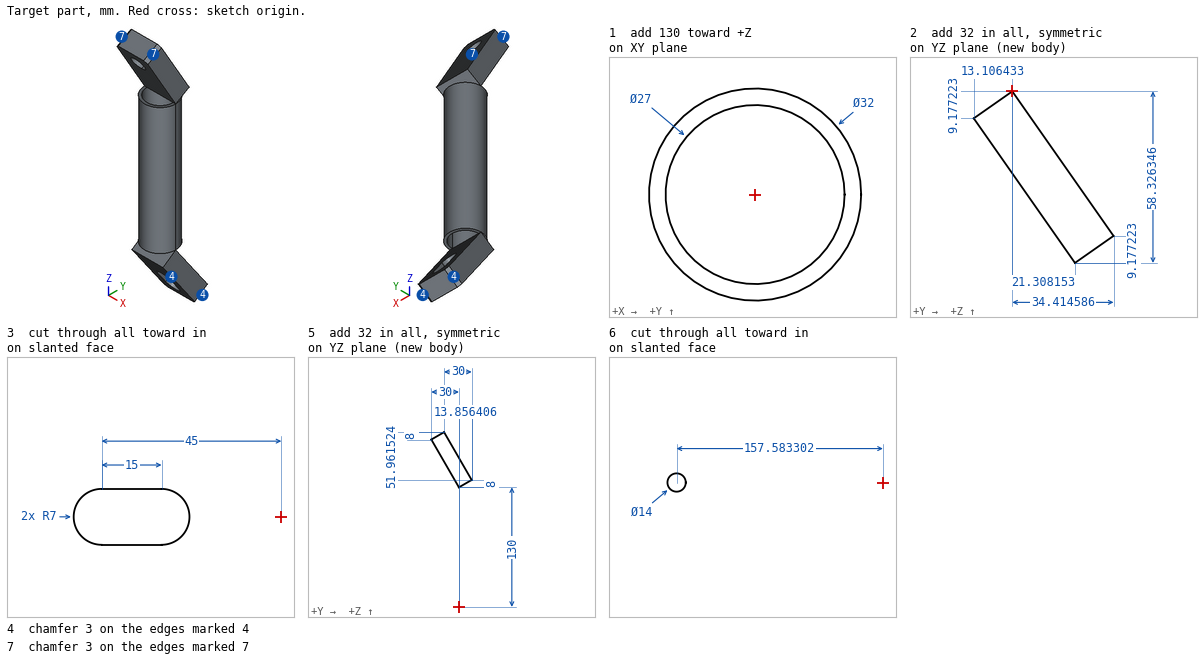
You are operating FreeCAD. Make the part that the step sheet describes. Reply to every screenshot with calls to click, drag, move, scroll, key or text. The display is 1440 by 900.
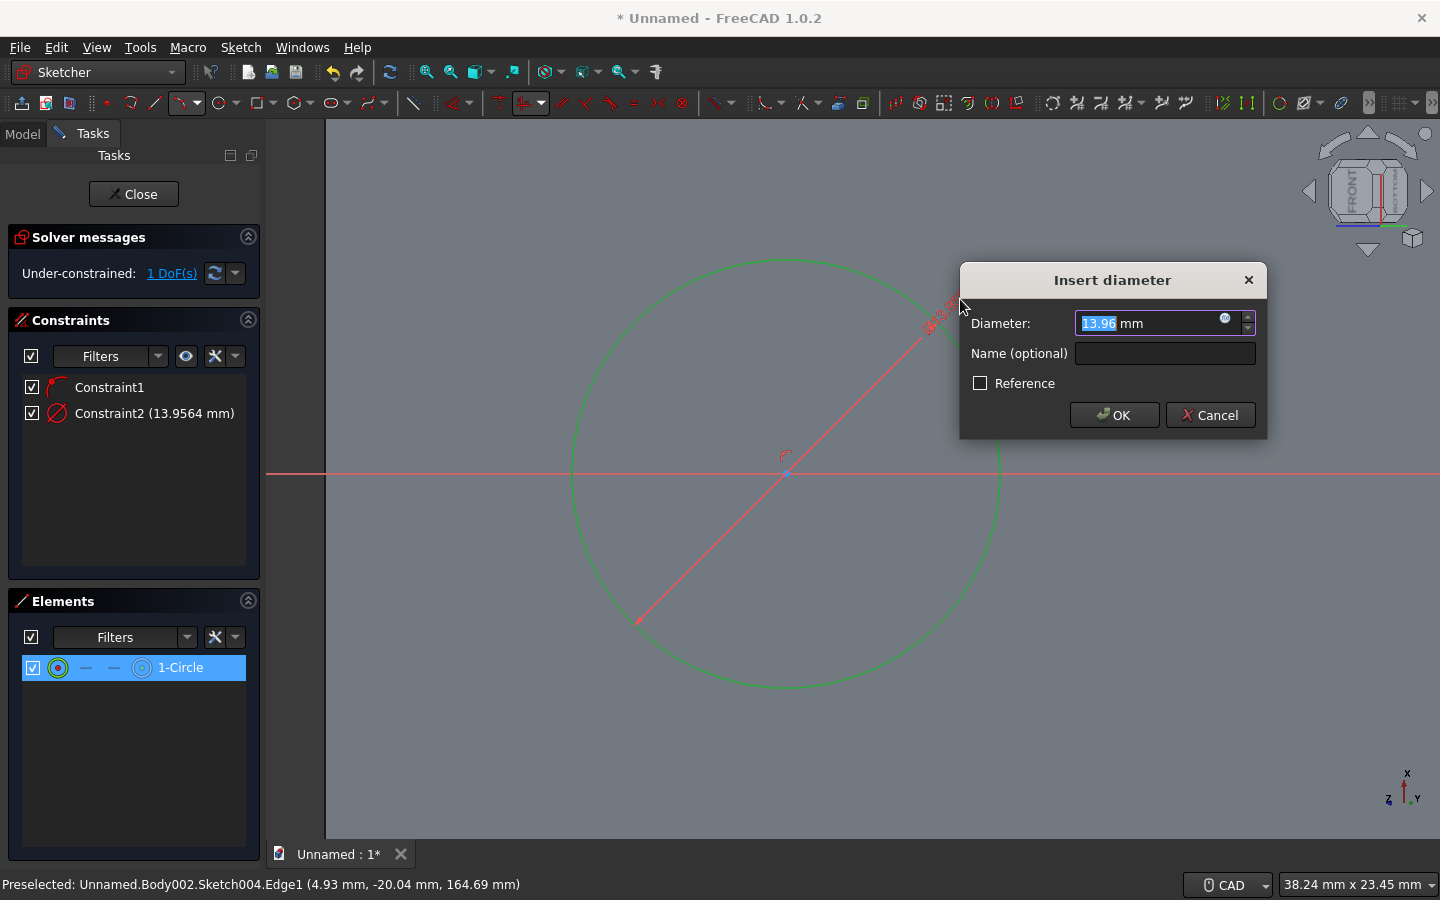
text(14)
key(Return)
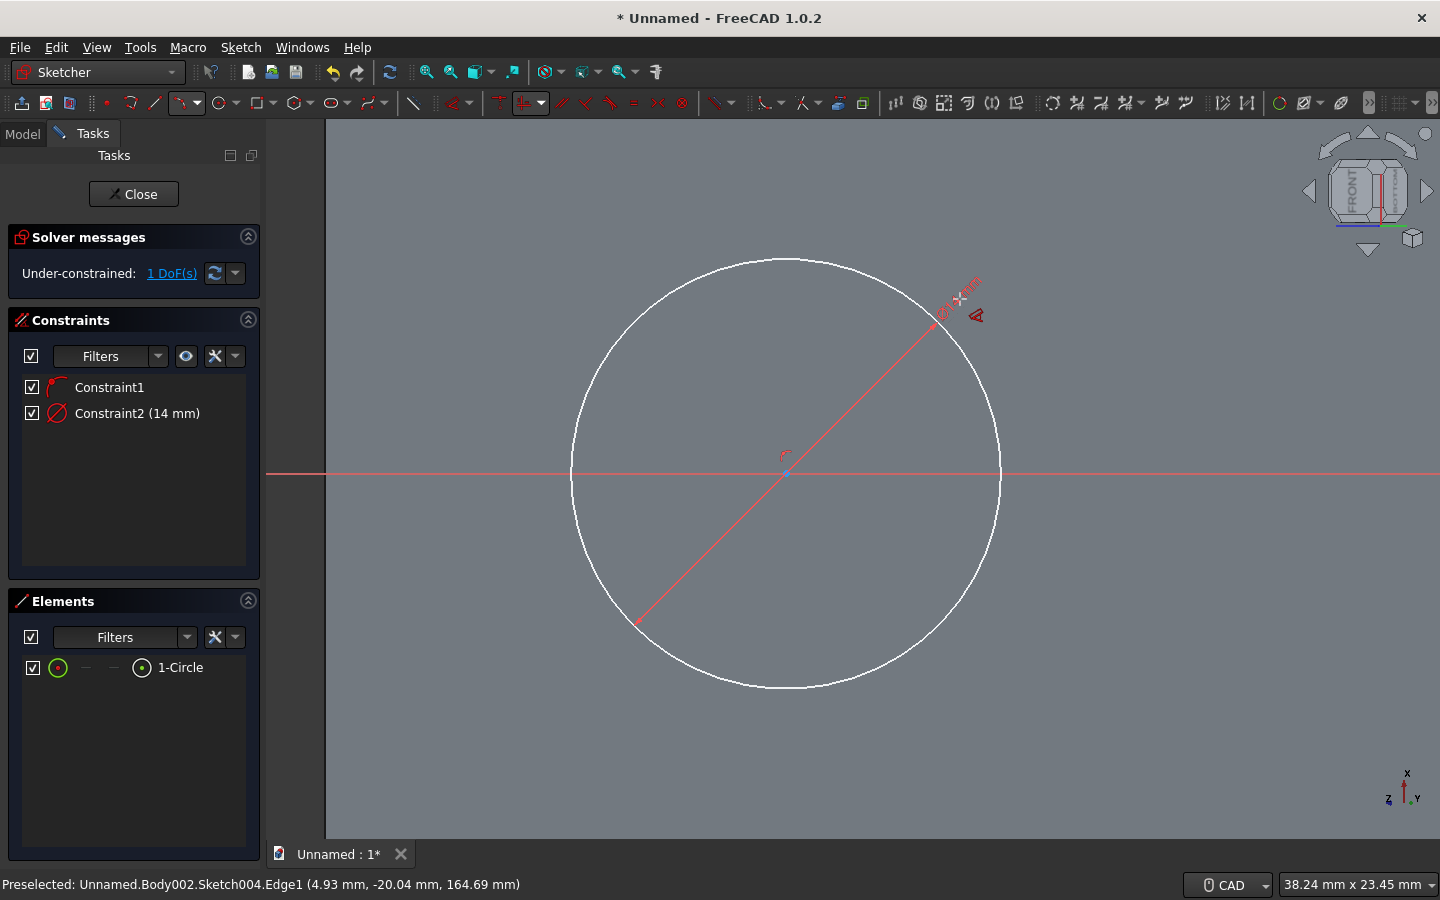
click(786, 474)
click(1031, 508)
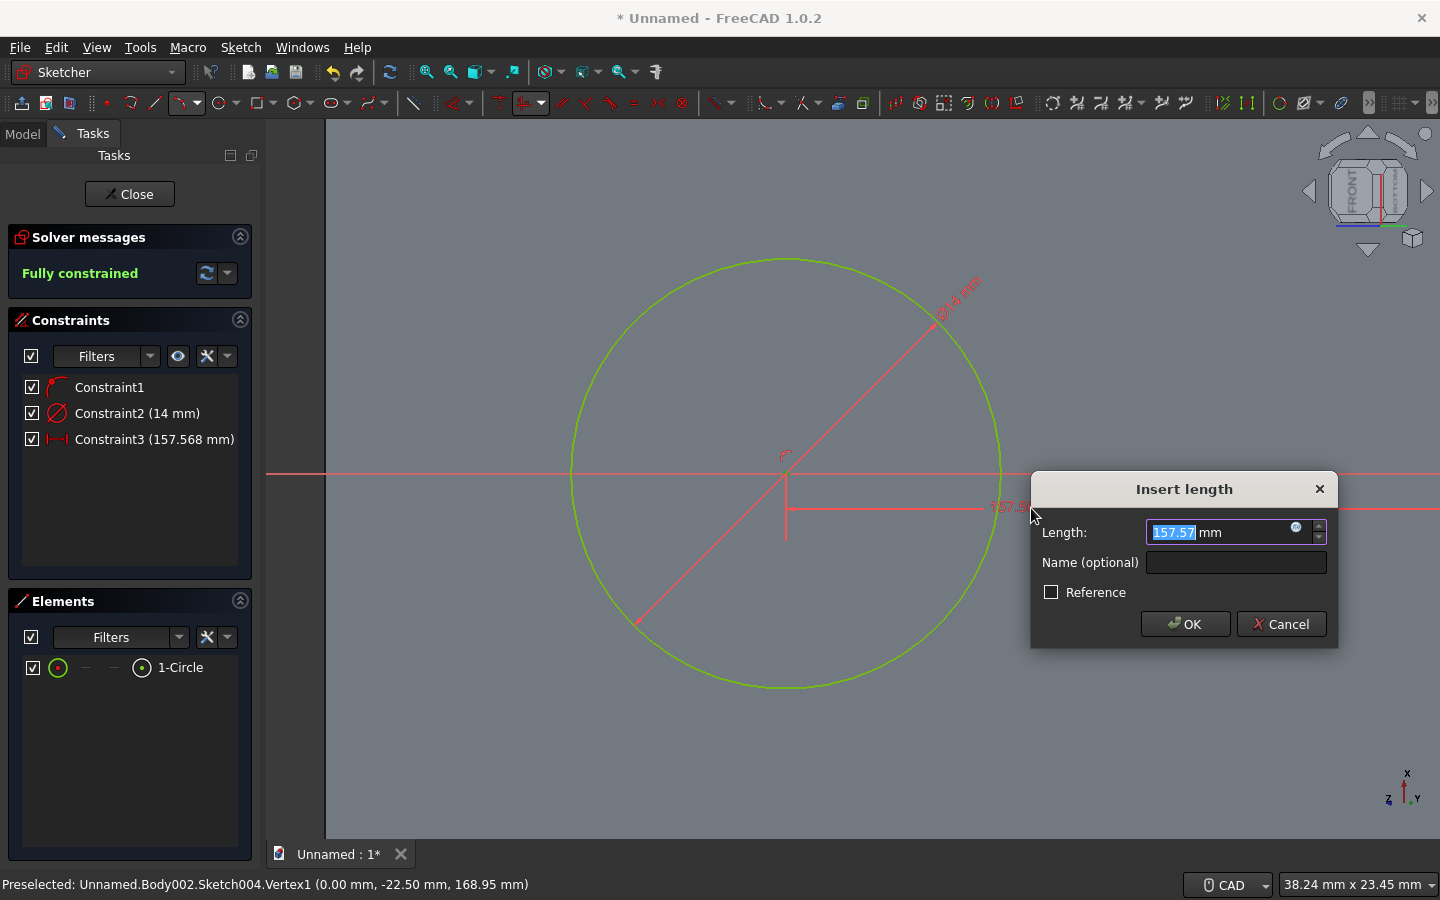
text(157.583302)
key(Return)
key(Escape)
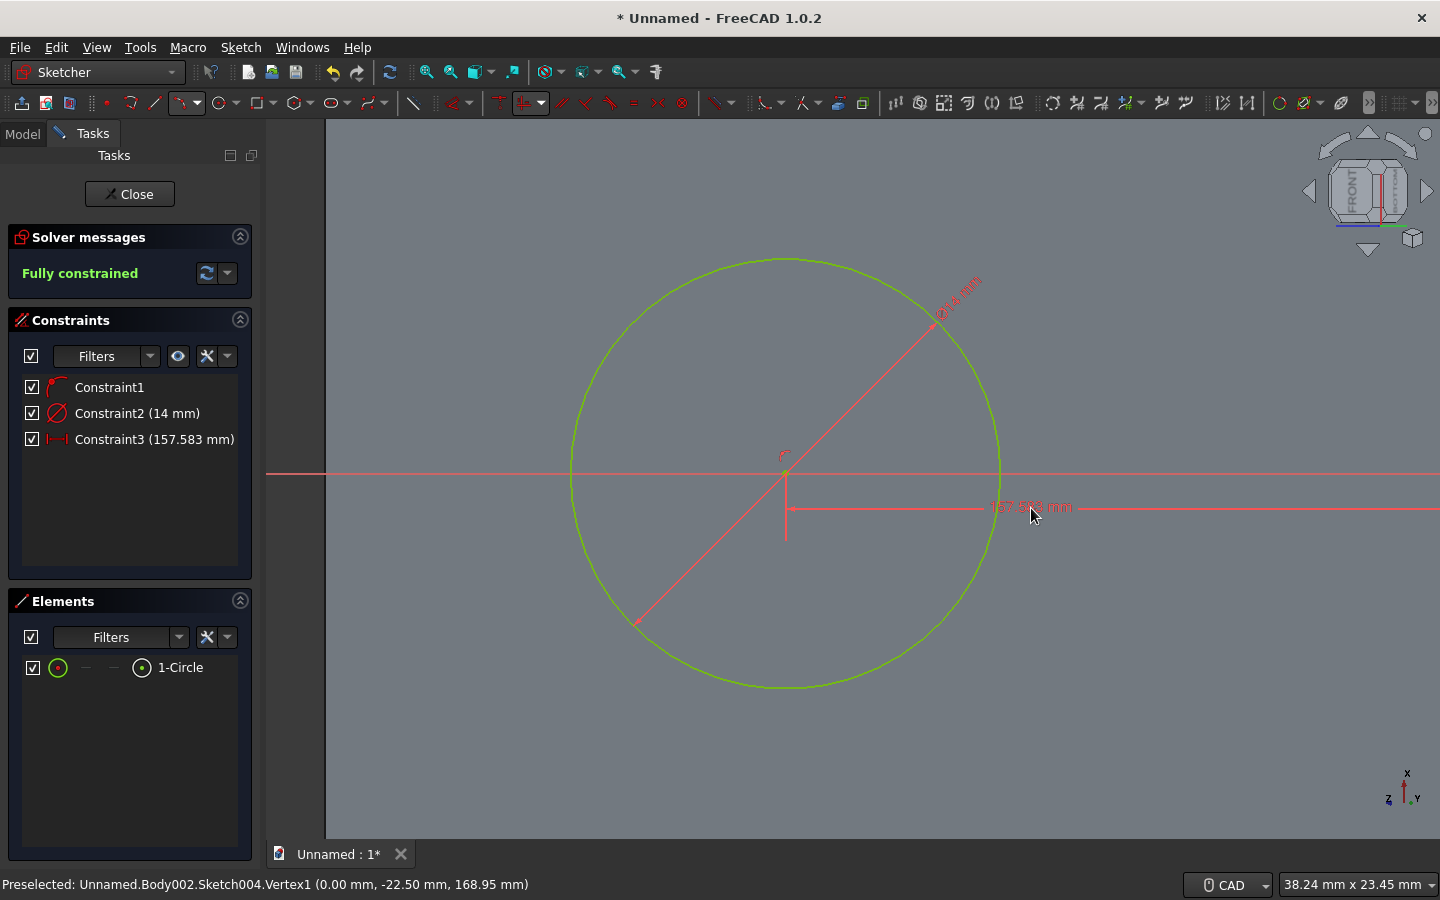
click(130, 194)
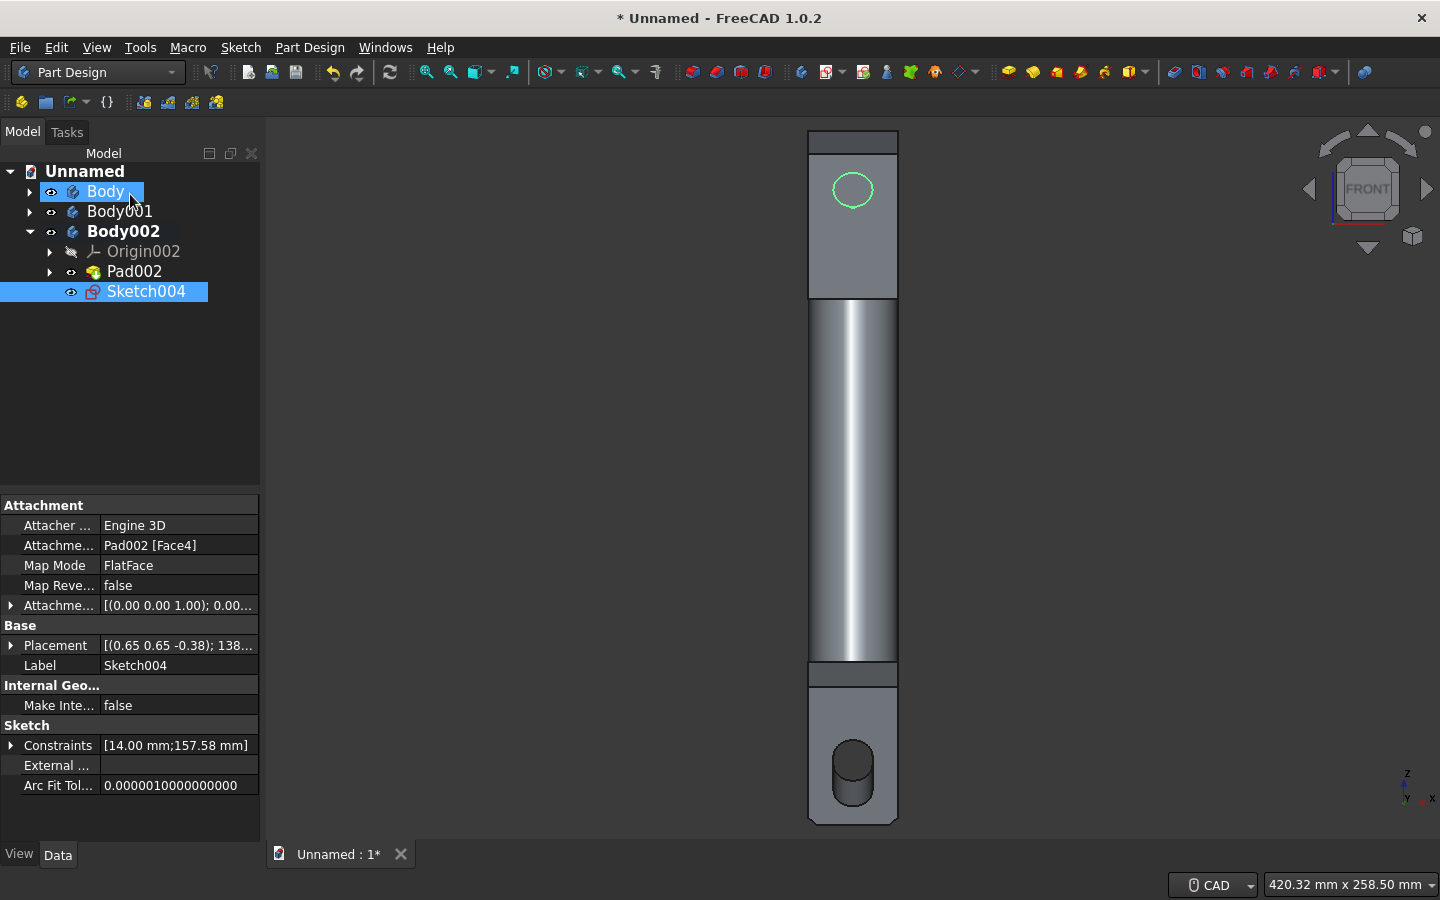
click(1176, 72)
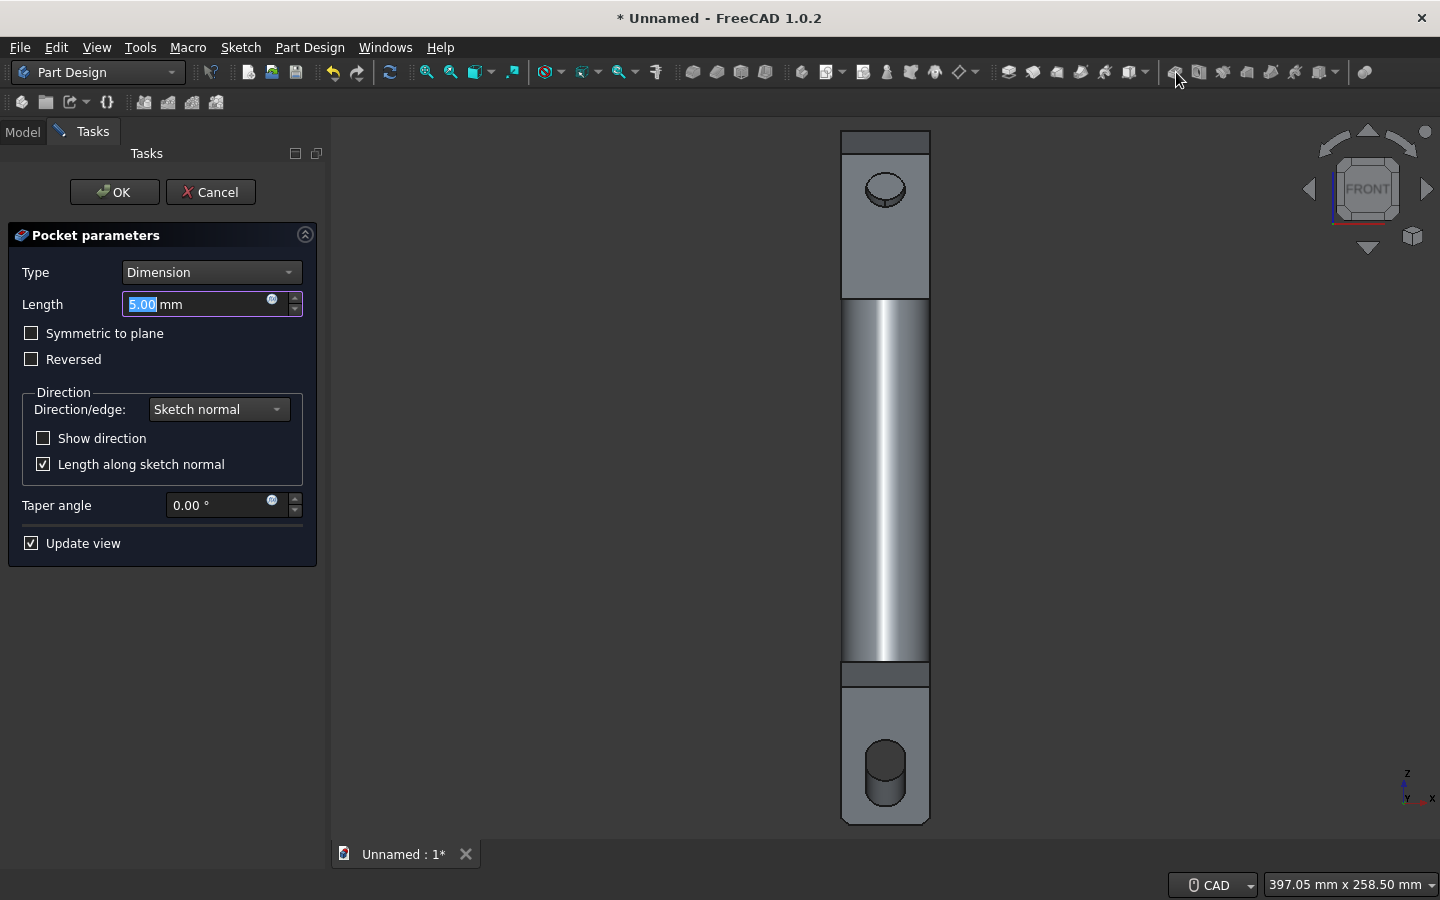
click(212, 272)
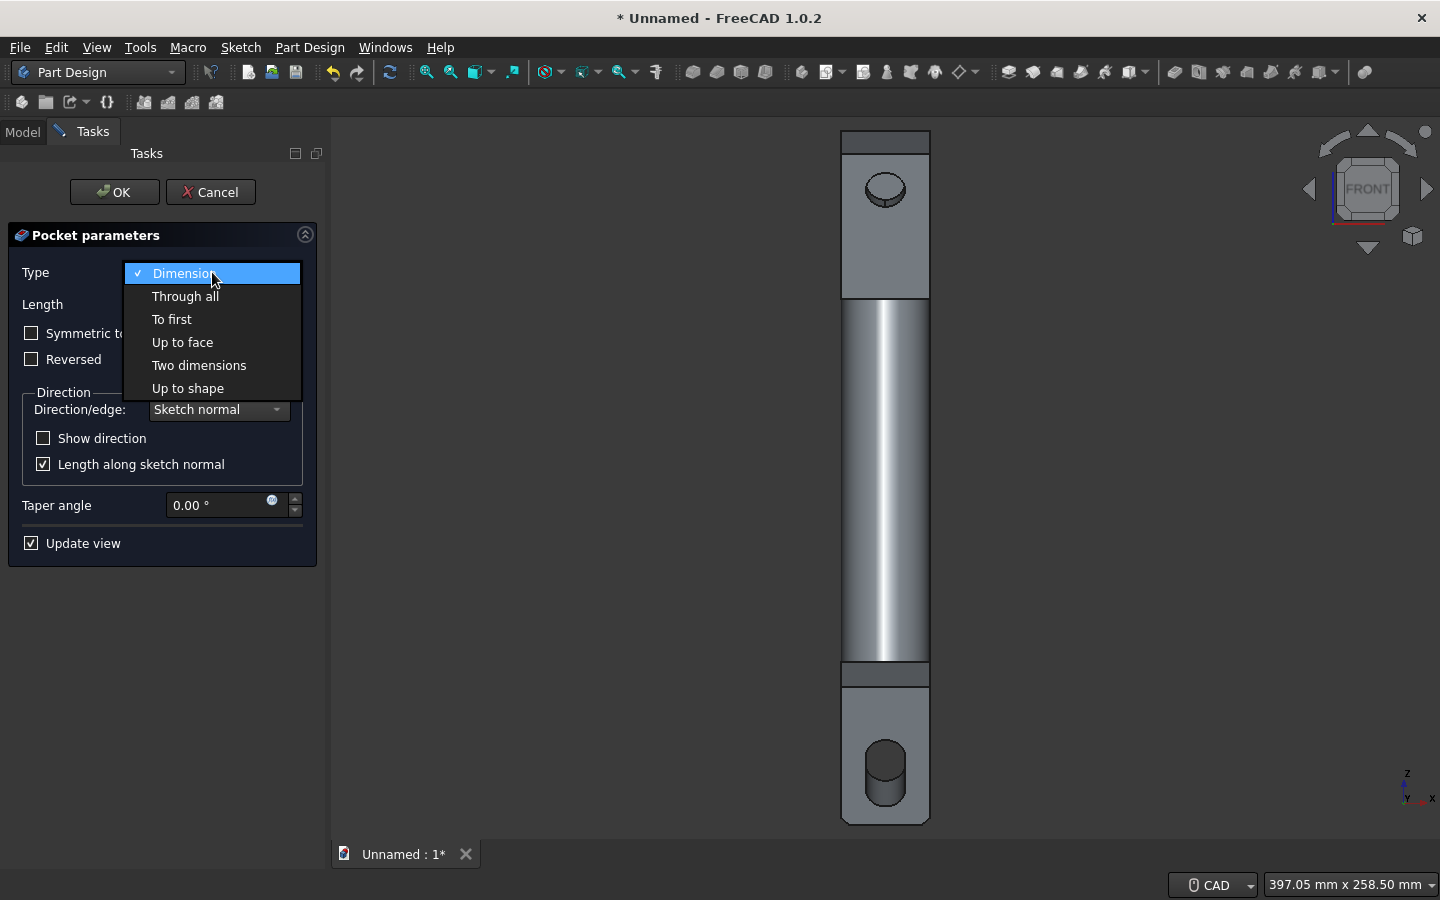
click(212, 296)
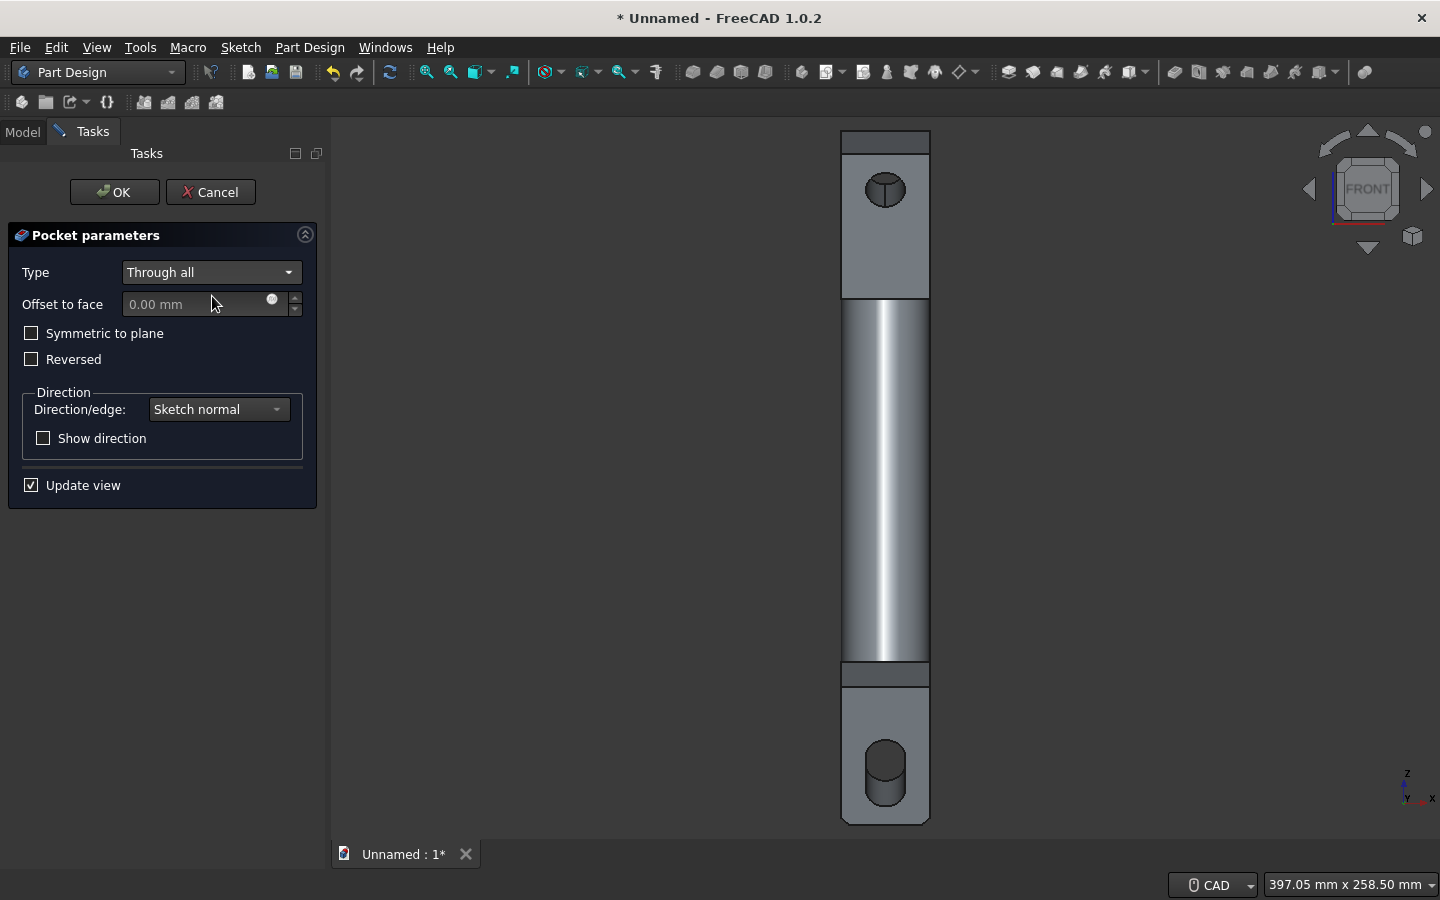
click(115, 192)